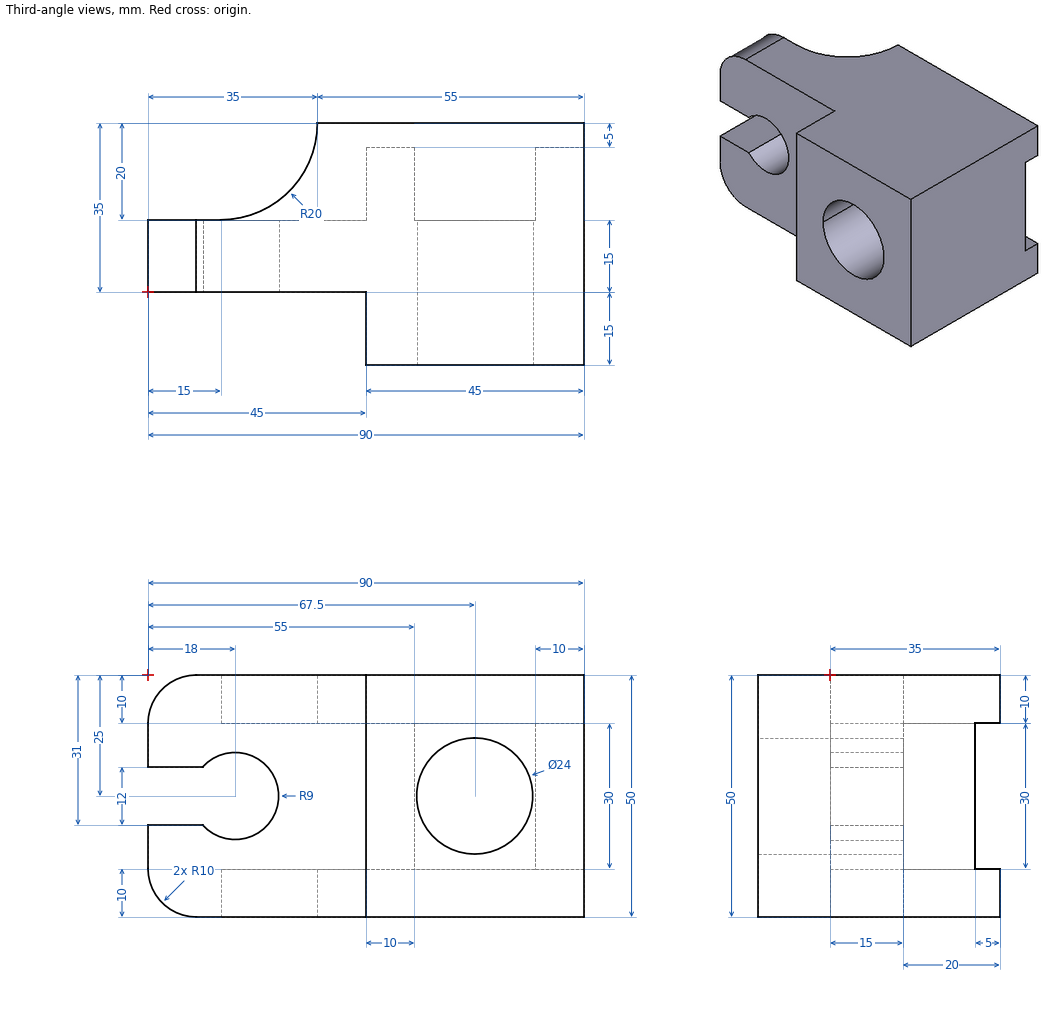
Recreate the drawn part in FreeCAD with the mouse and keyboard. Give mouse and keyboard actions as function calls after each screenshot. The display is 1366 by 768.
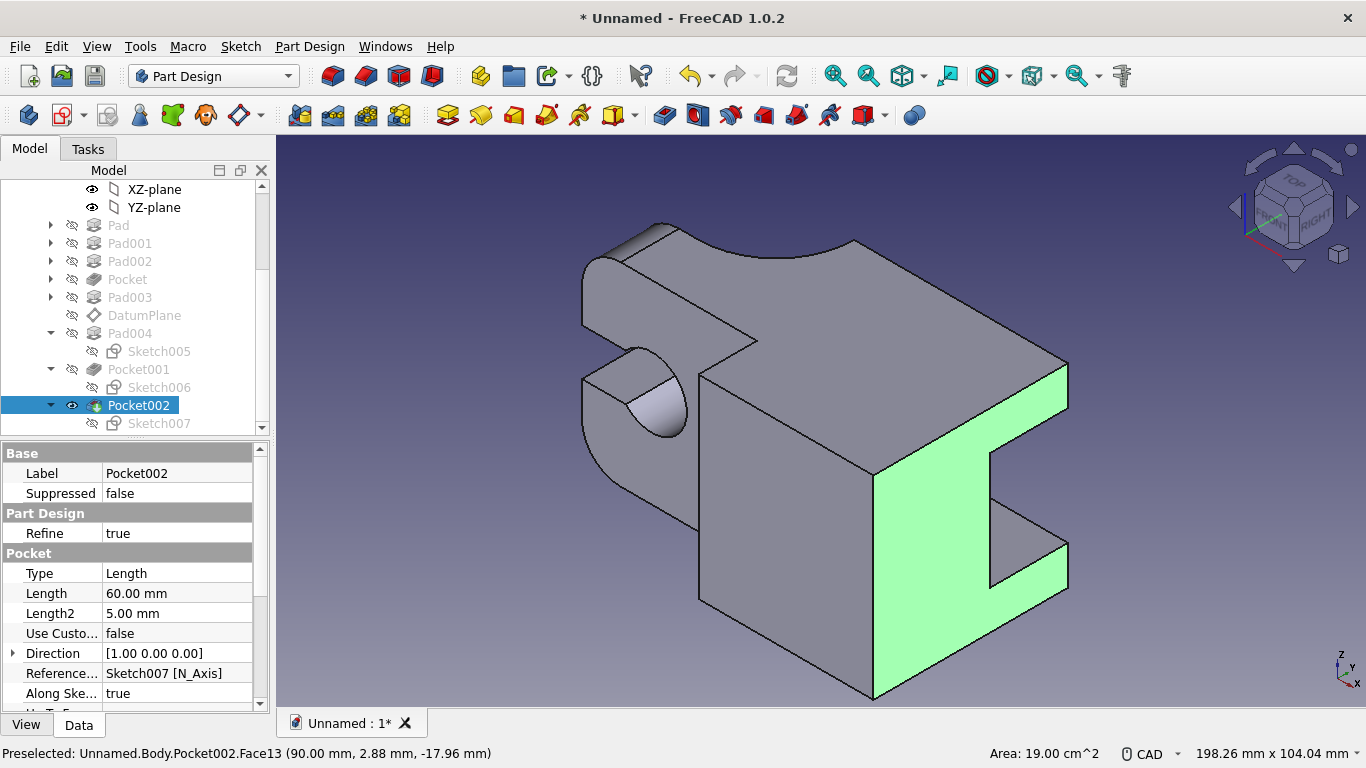
click(62, 116)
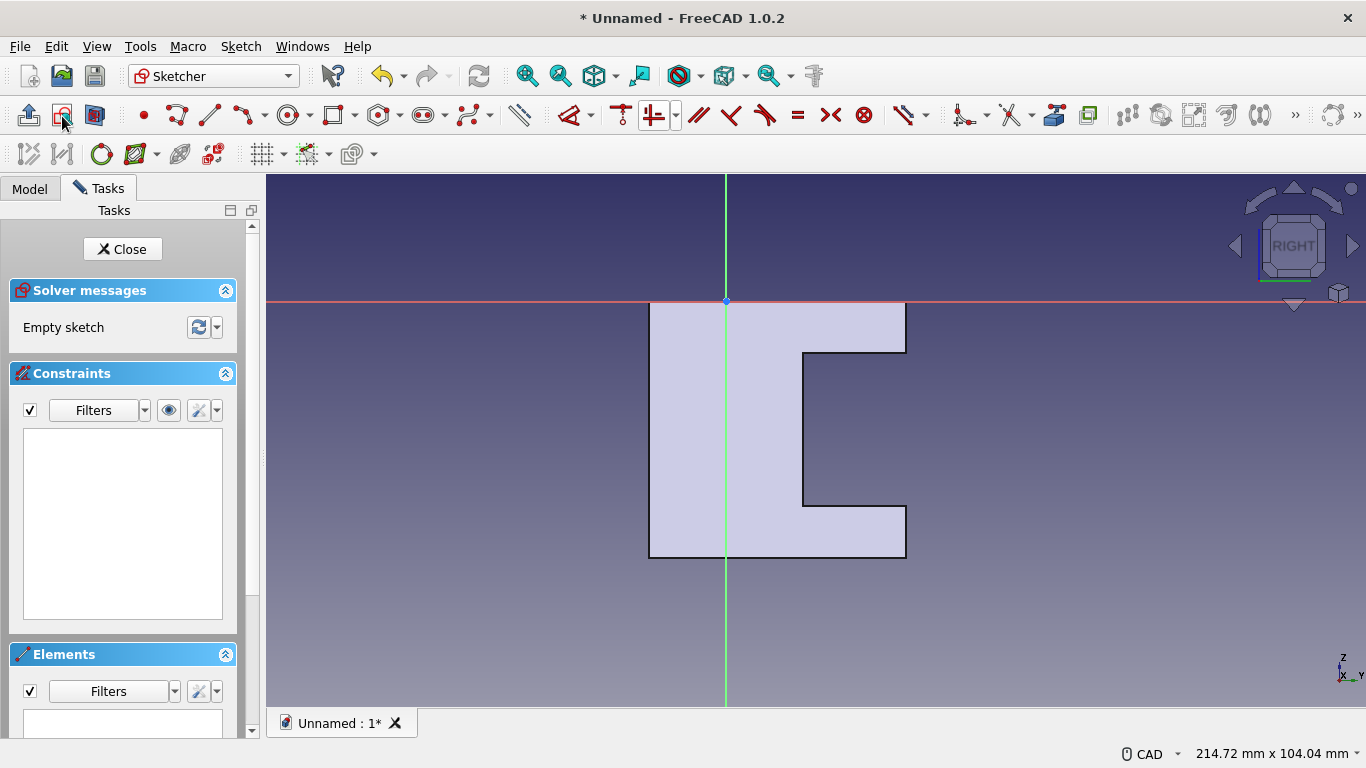
scroll(955, 330, up, 2)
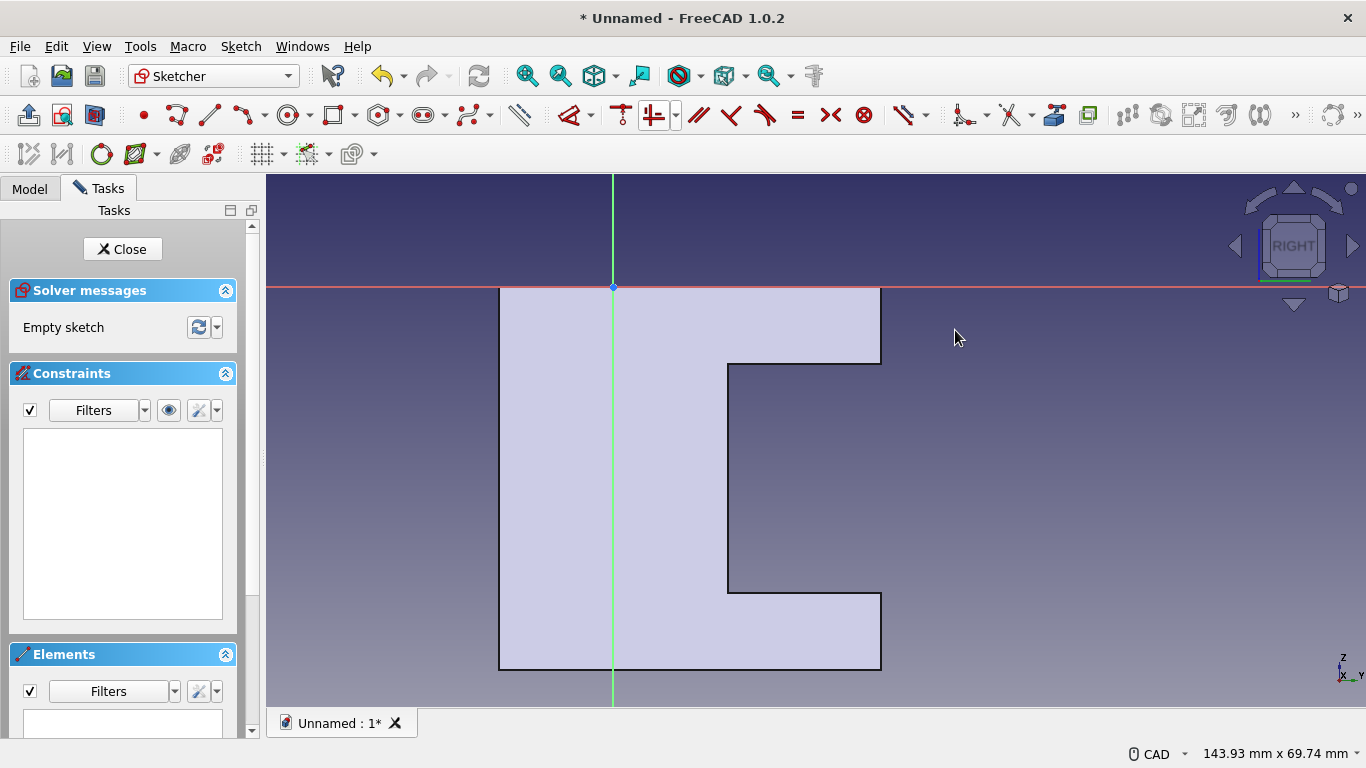
click(332, 116)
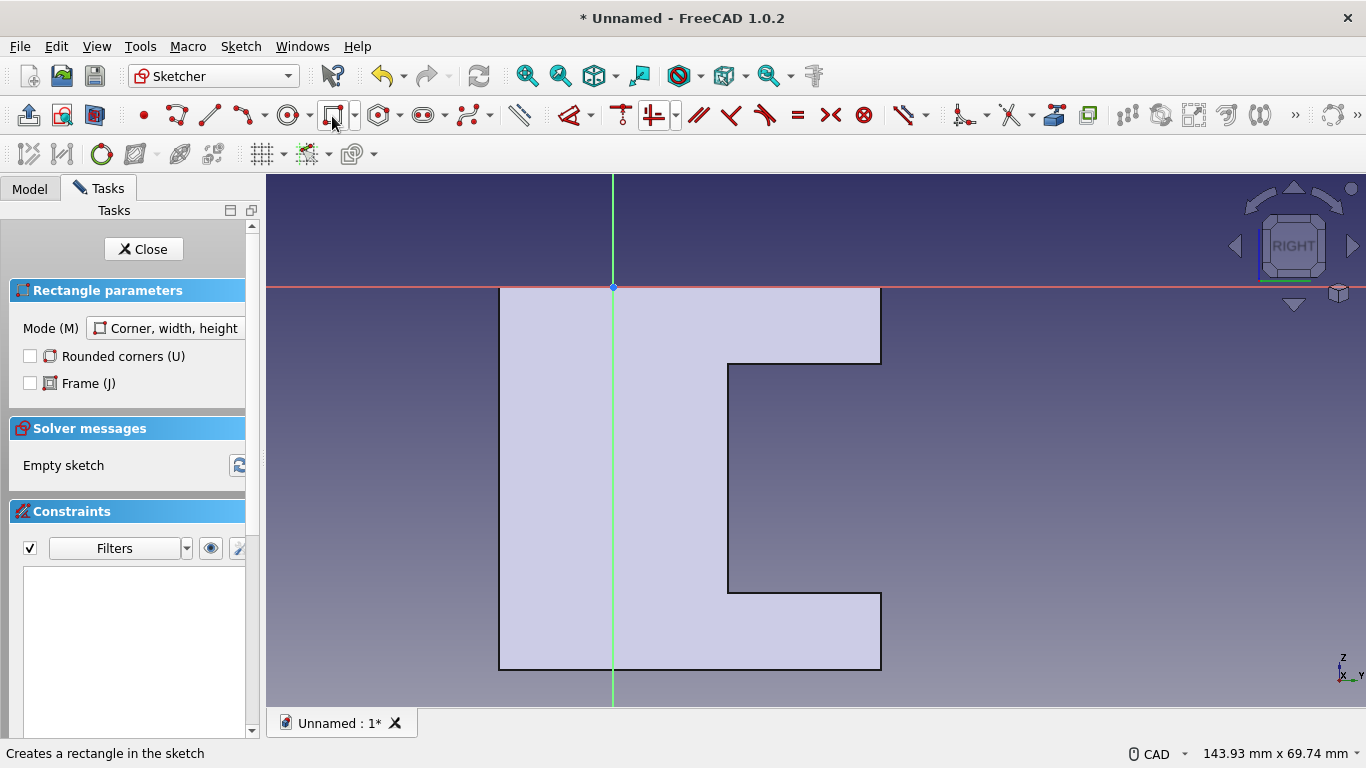
click(728, 364)
click(881, 593)
key(Escape)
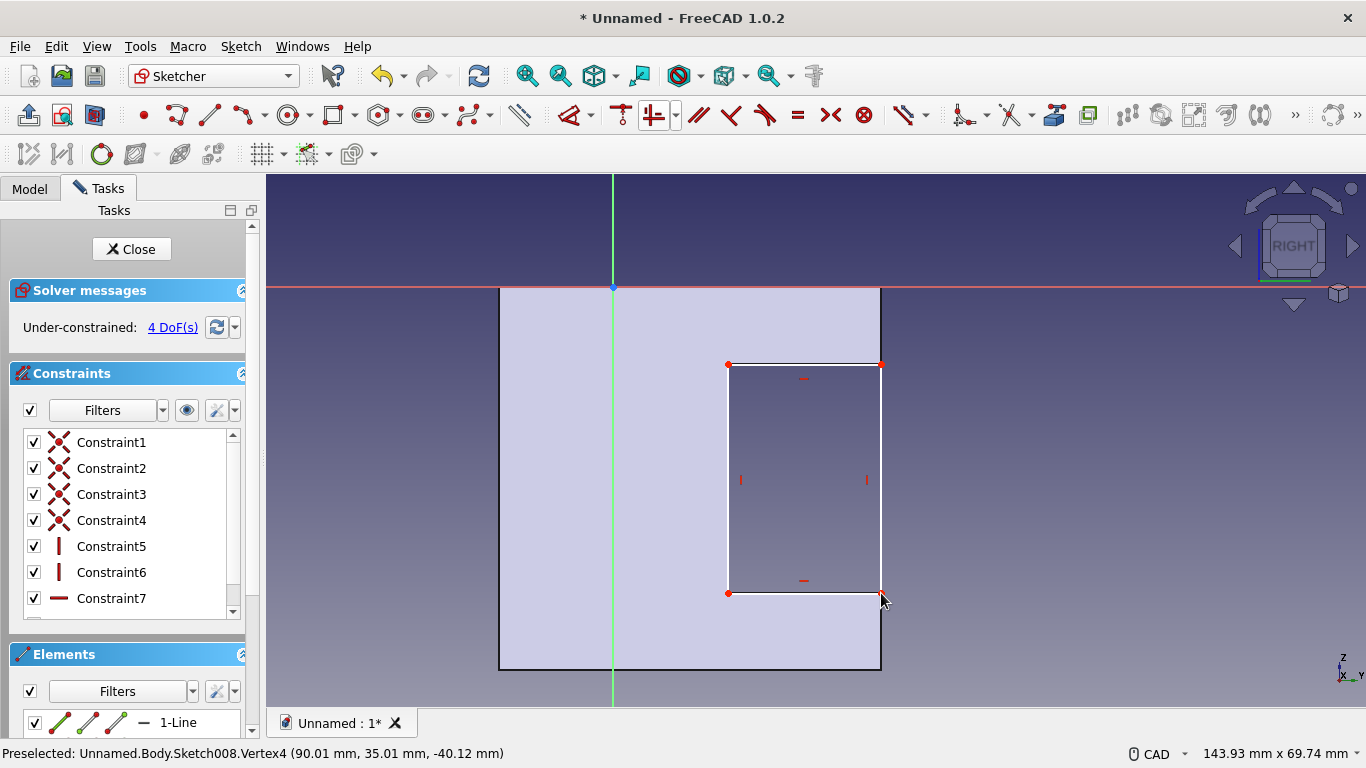
key(d)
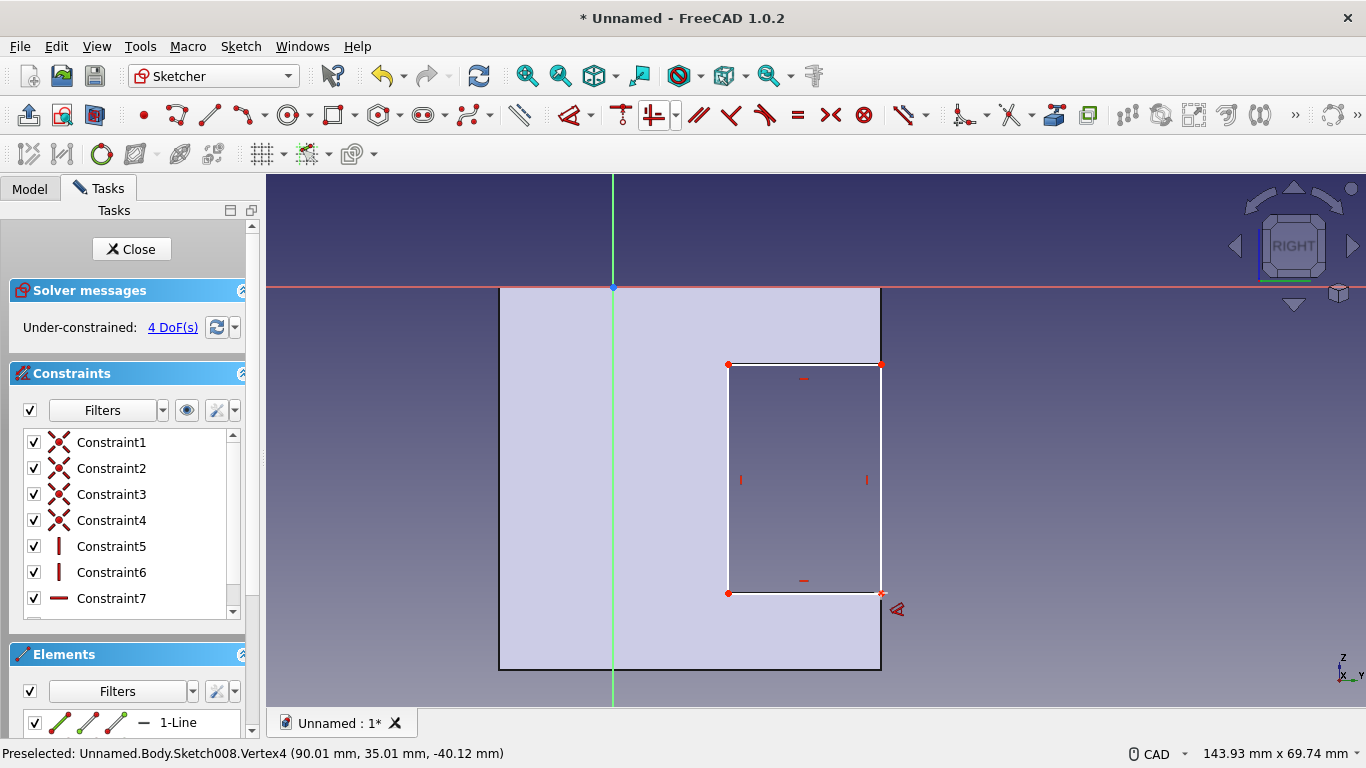
click(728, 434)
click(694, 479)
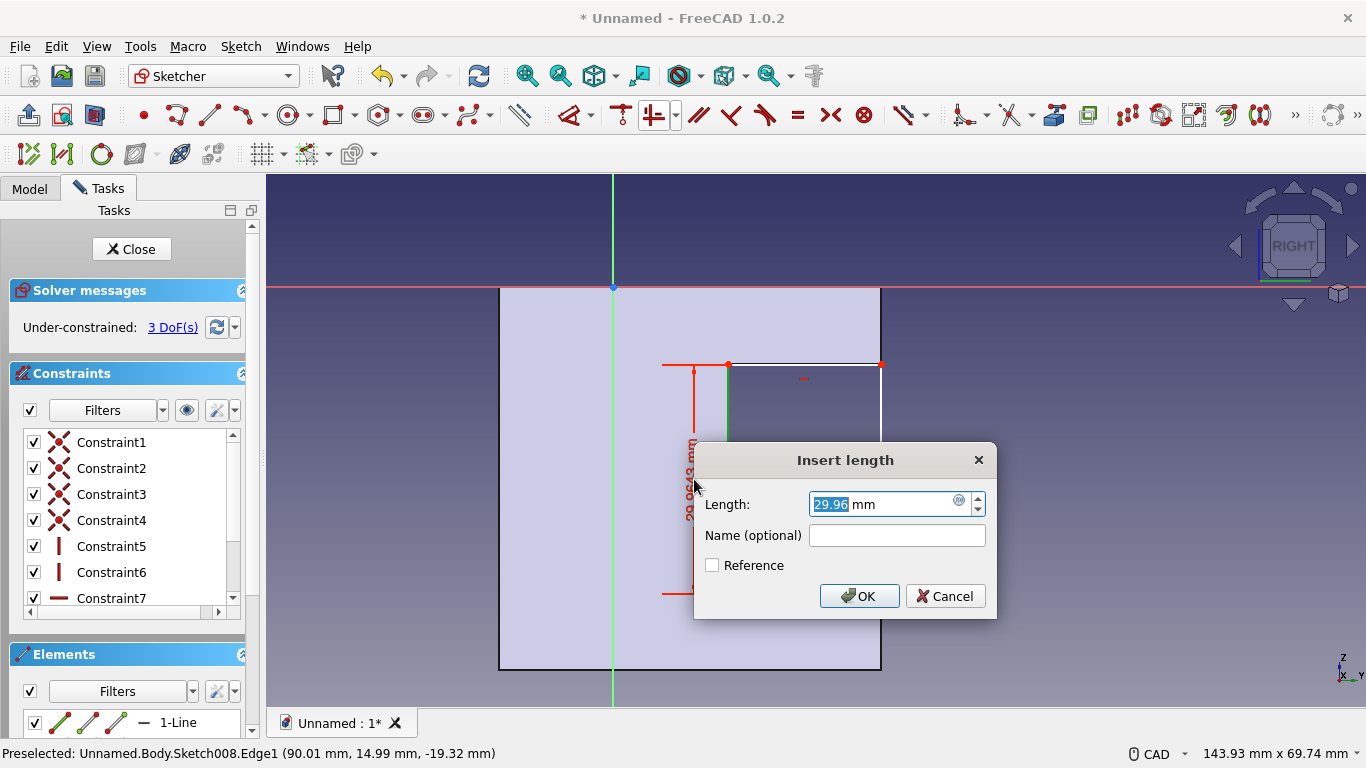
text(30)
key(Return)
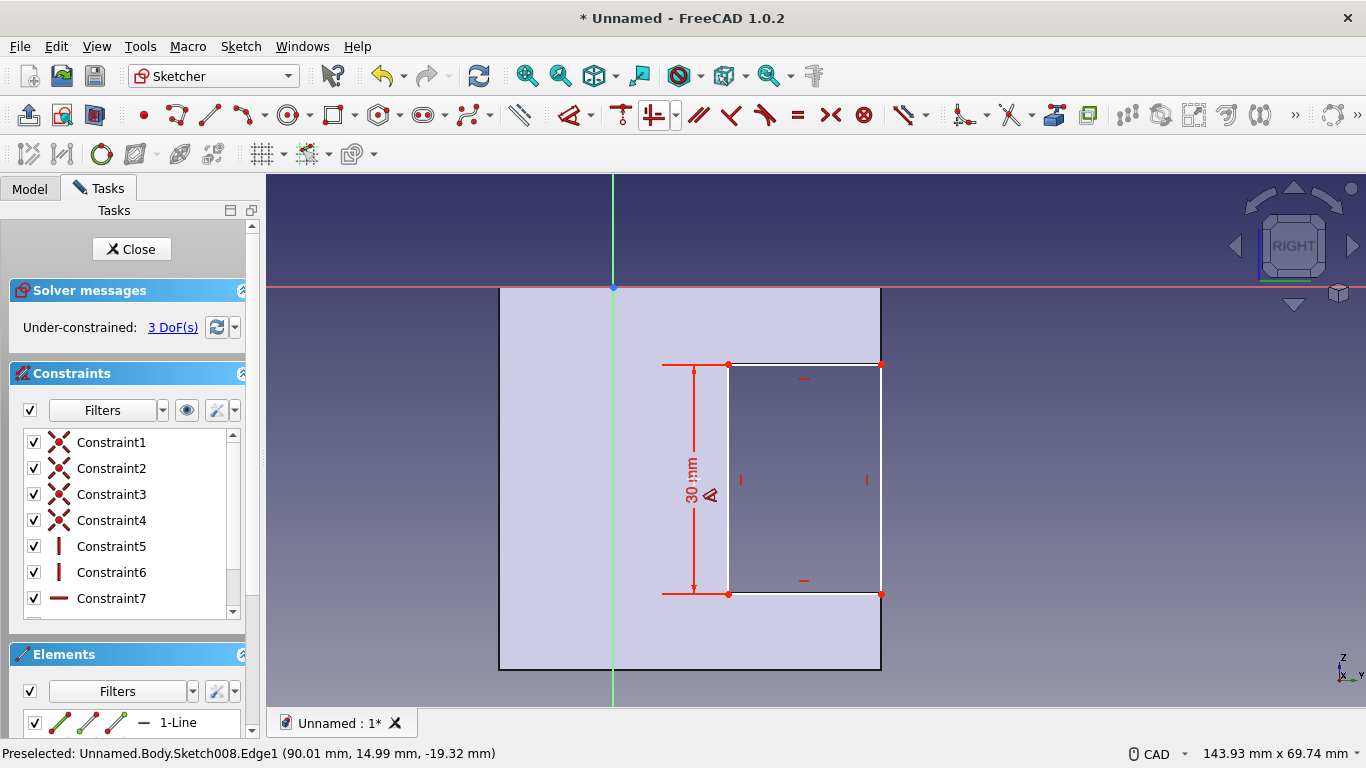
click(774, 594)
click(805, 628)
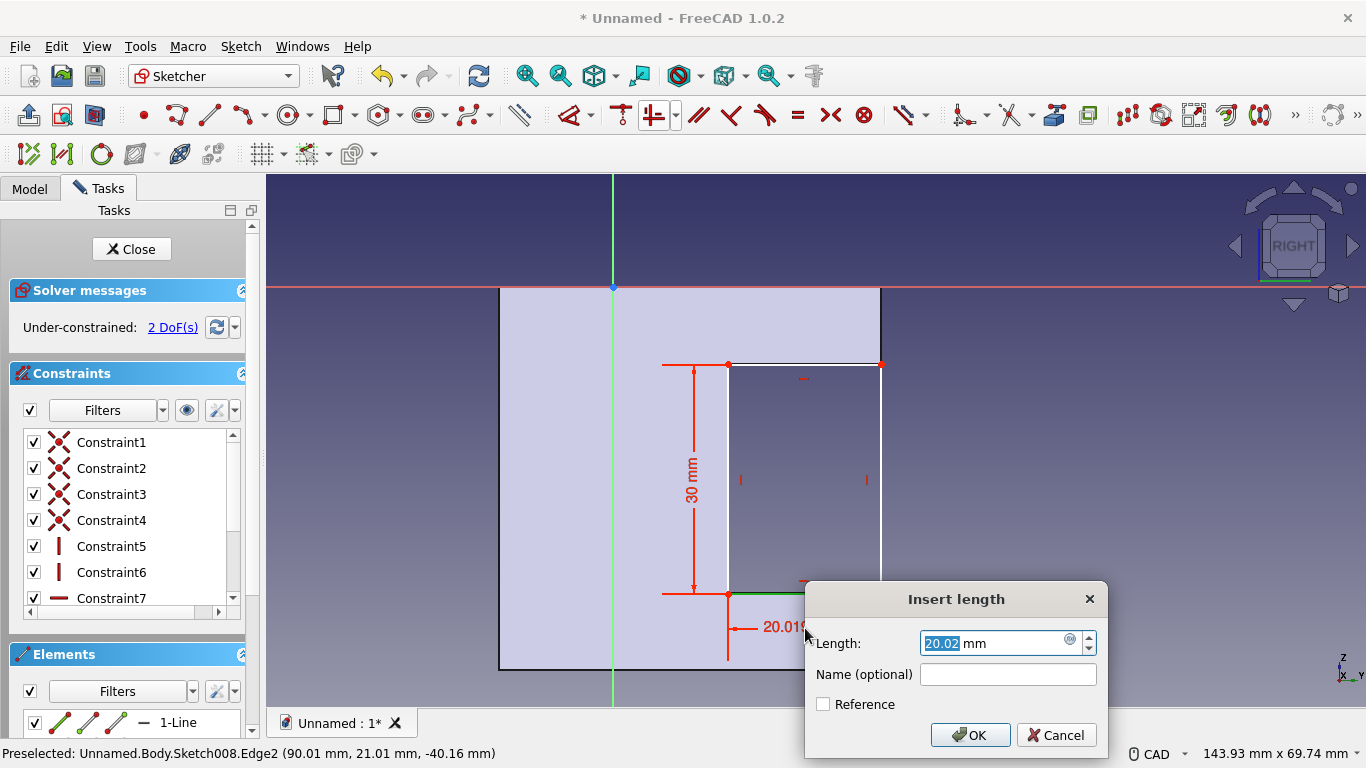
text(20)
key(Return)